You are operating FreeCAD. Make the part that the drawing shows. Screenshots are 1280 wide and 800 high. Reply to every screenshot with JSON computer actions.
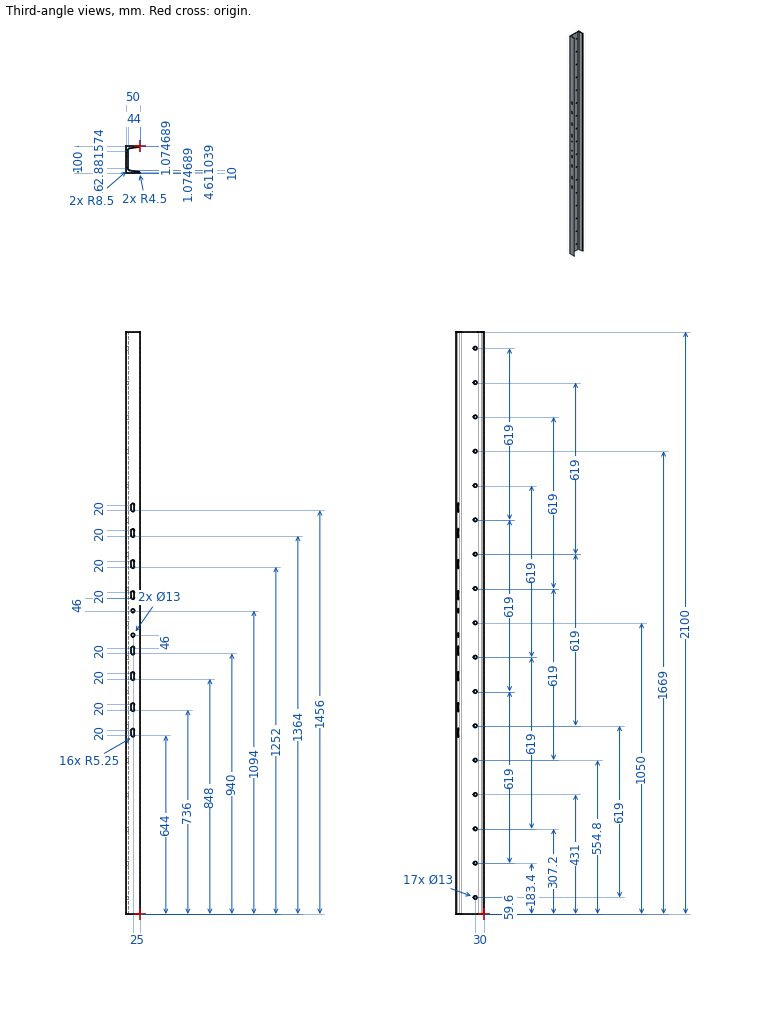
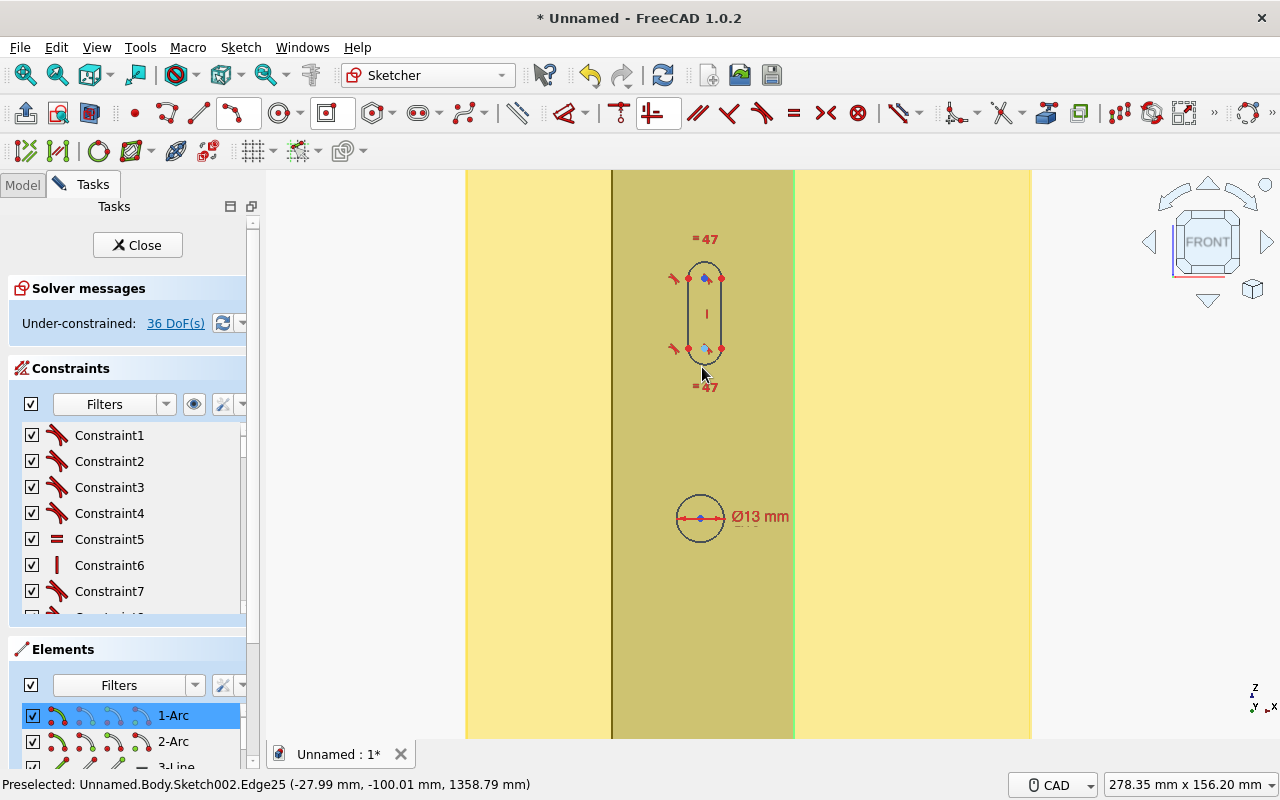
{"action": "left_click", "coordinate": [695, 361]}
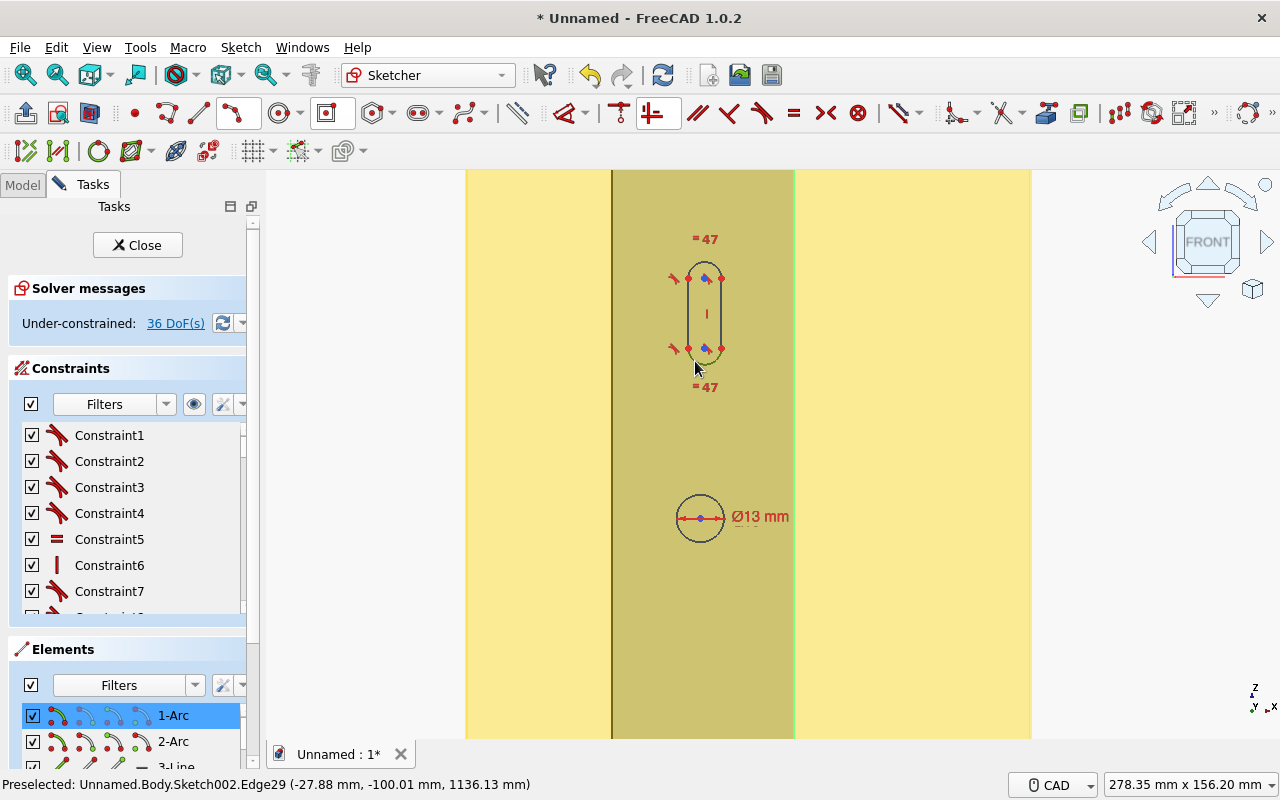
{"action": "left_click", "coordinate": [794, 114]}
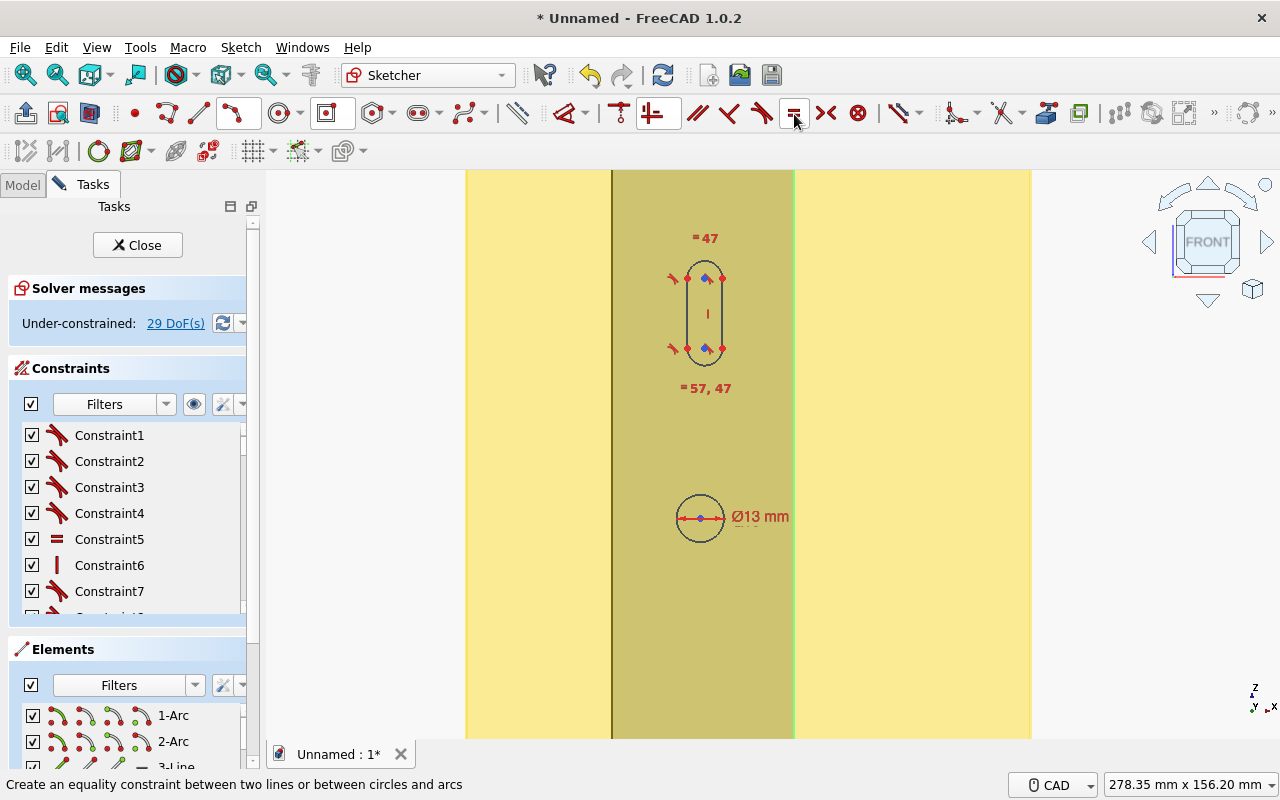
{"action": "left_click", "coordinate": [564, 114]}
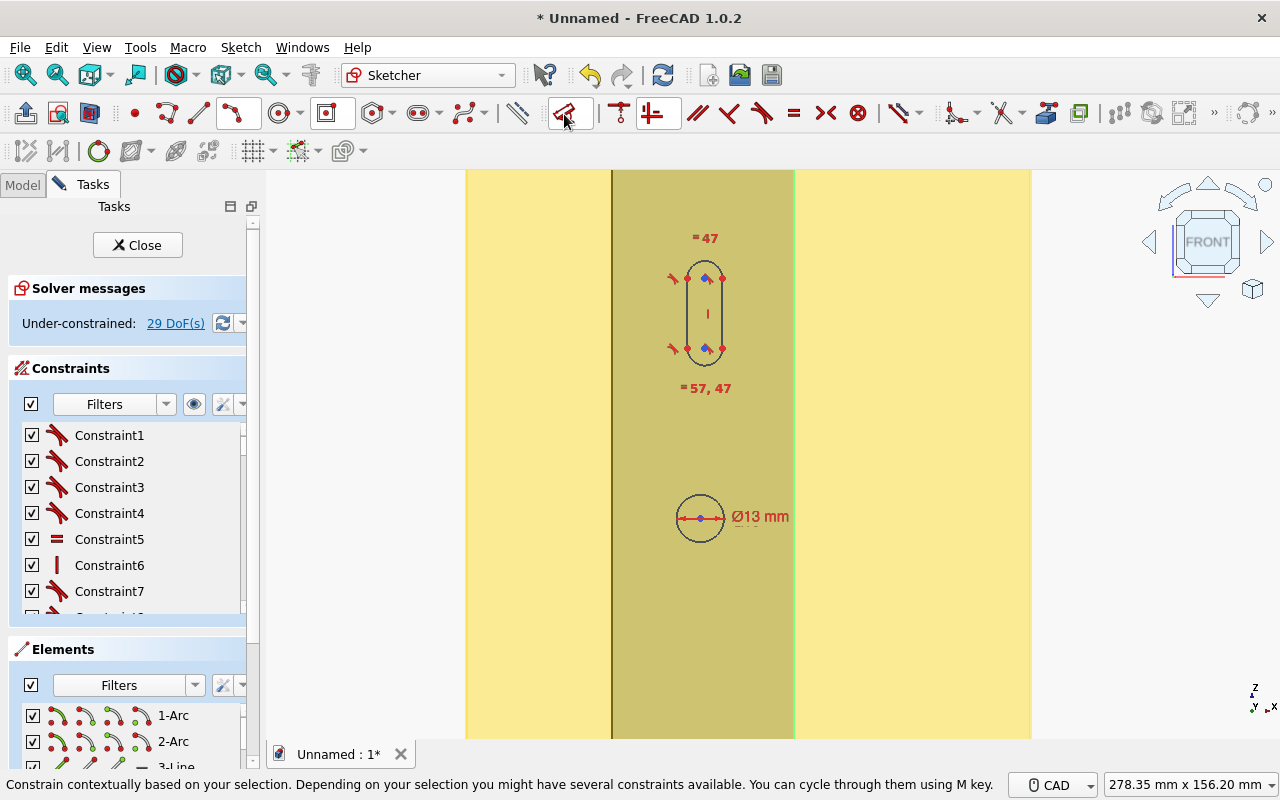
{"action": "scroll", "coordinate": [702, 367], "scroll_direction": "down", "scroll_amount": 14}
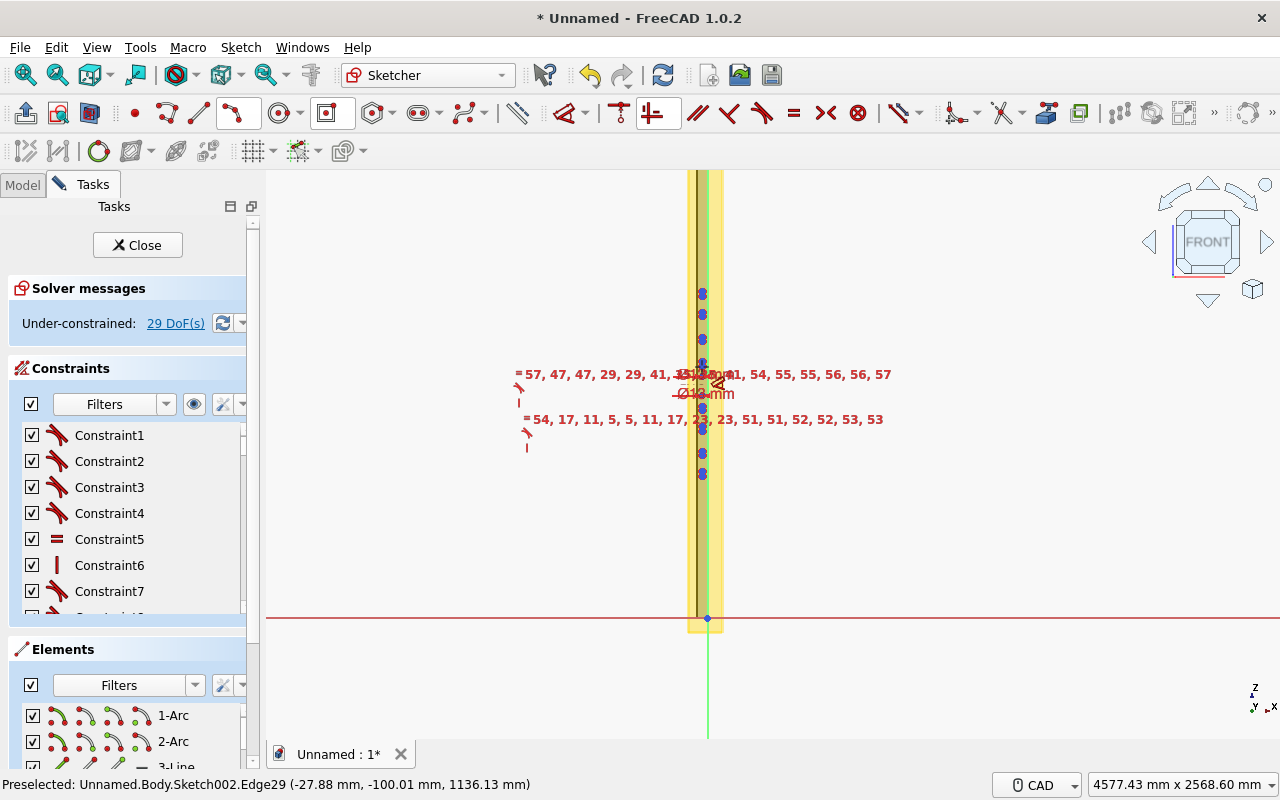
{"action": "scroll", "coordinate": [702, 477], "scroll_direction": "up", "scroll_amount": 18}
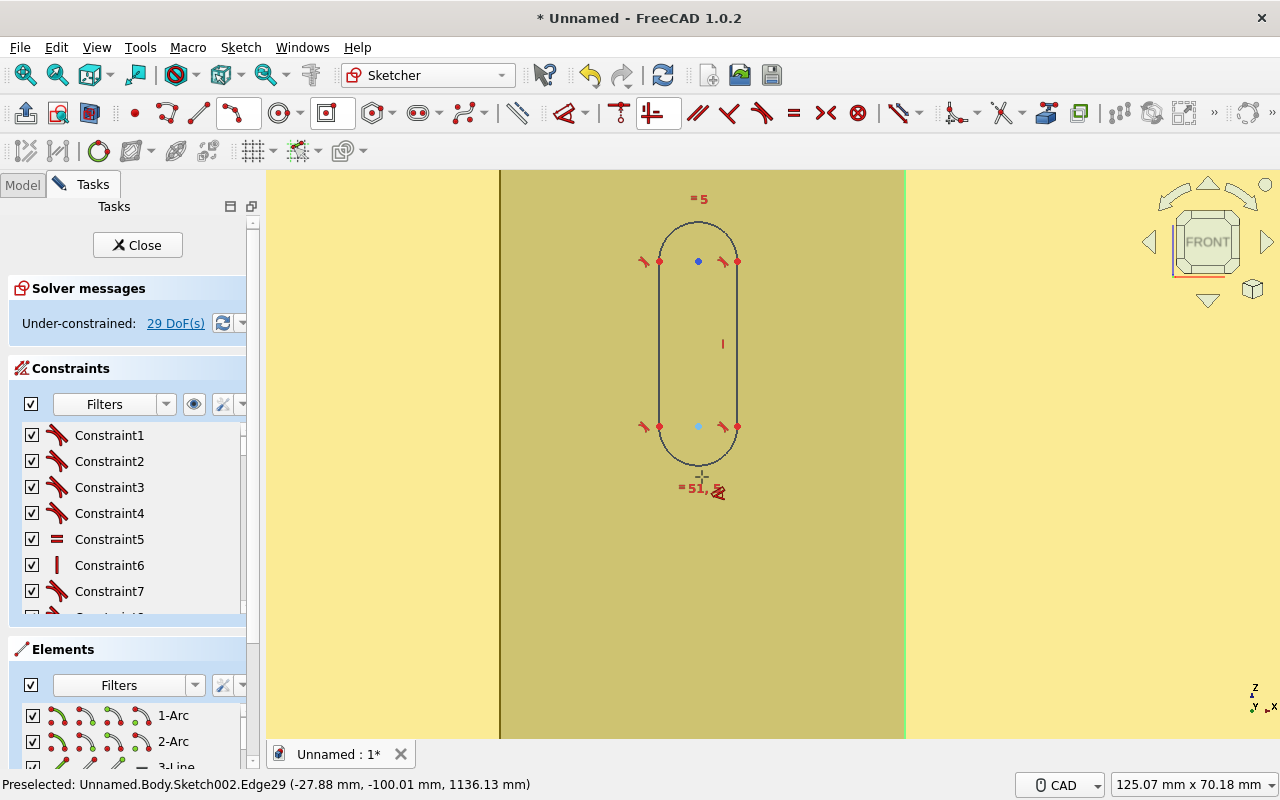
{"action": "left_click", "coordinate": [675, 458]}
{"action": "left_click", "coordinate": [656, 484]}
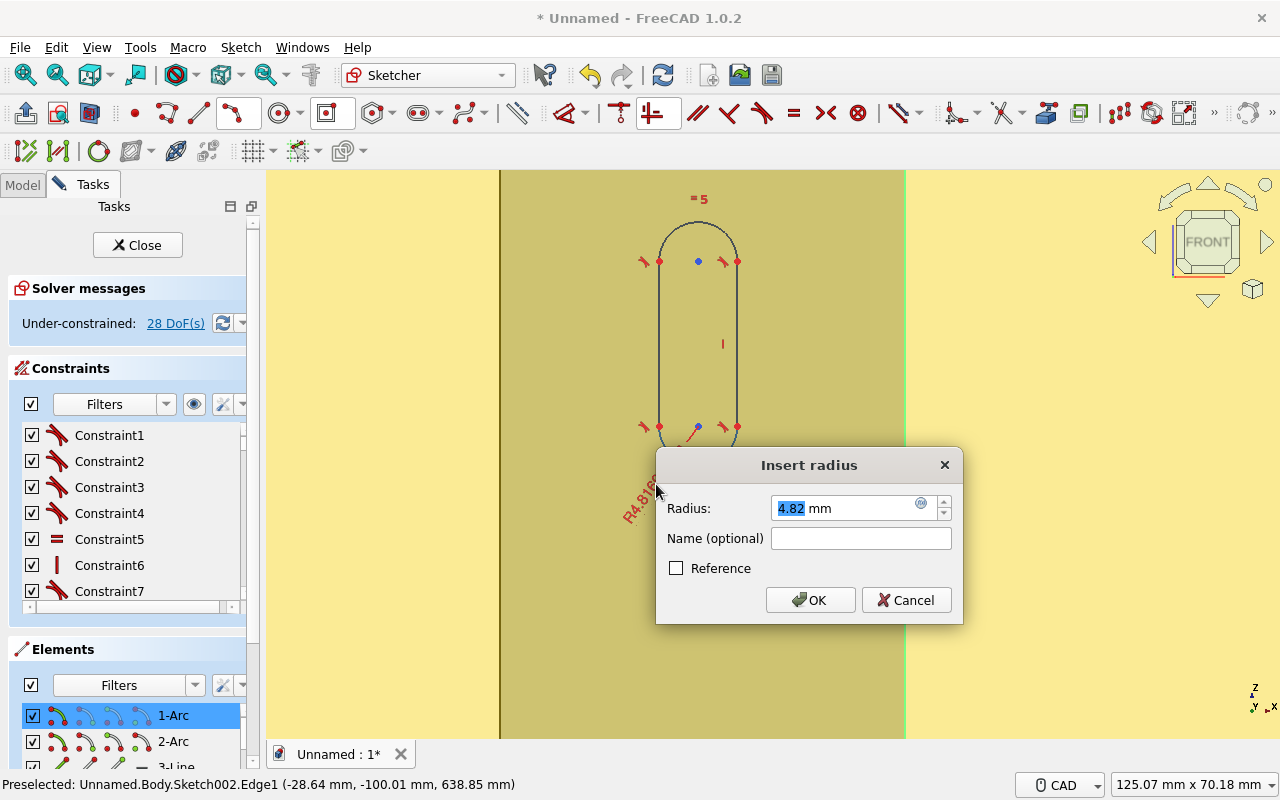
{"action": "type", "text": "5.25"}
{"action": "key", "text": "Return"}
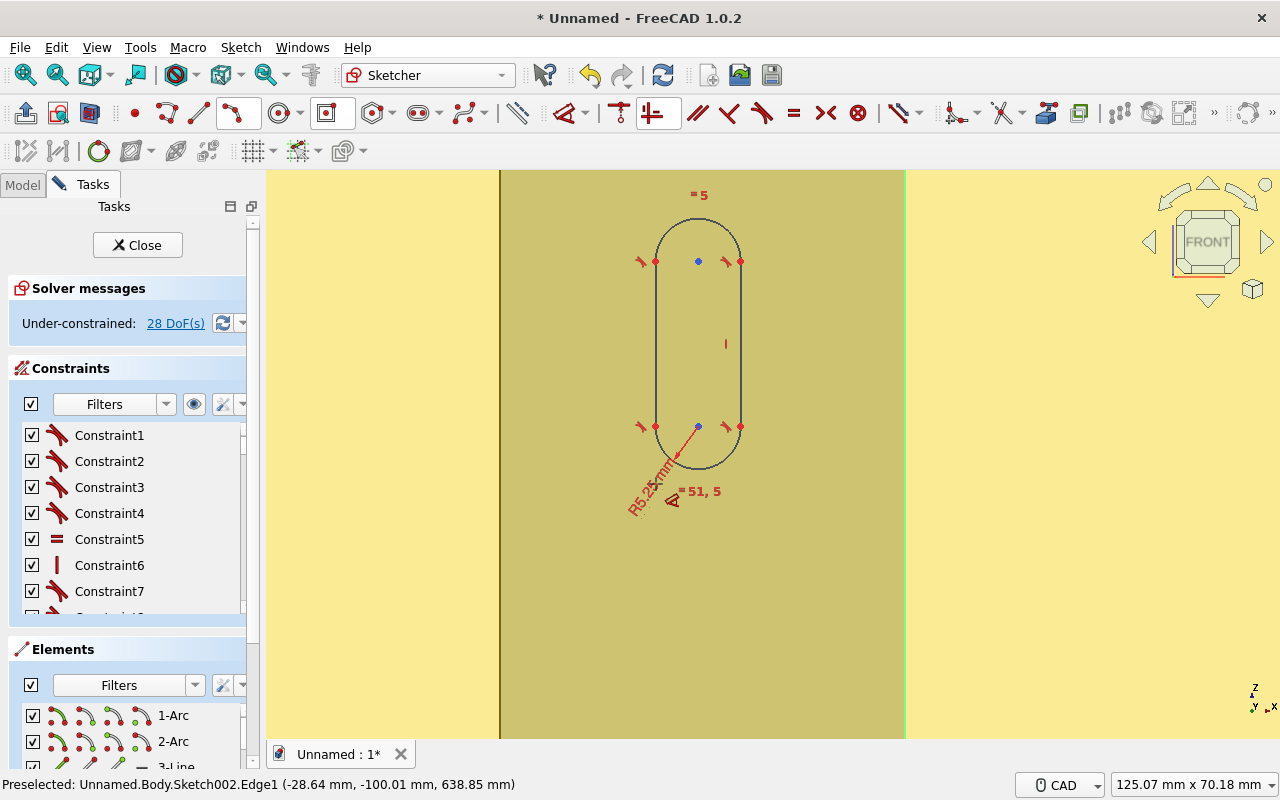
{"action": "scroll", "coordinate": [702, 483], "scroll_direction": "down", "scroll_amount": 17}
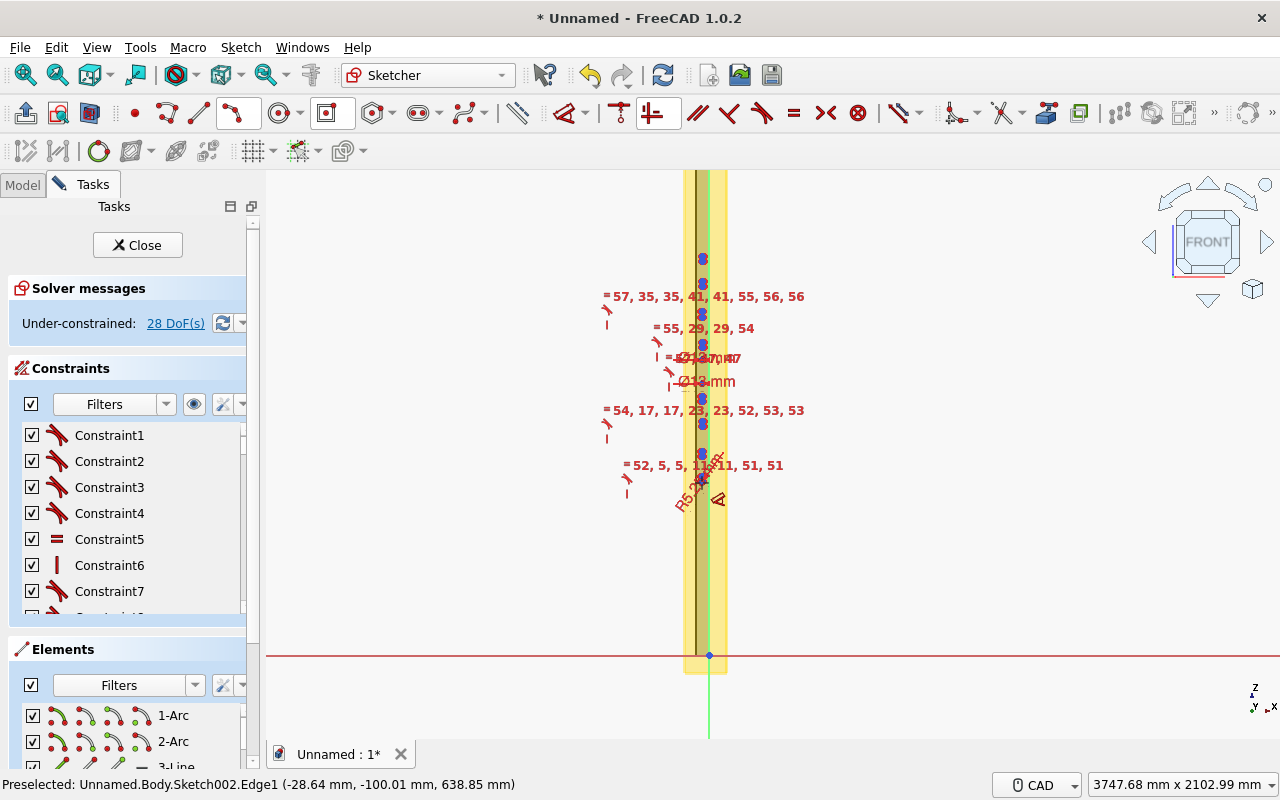
{"action": "scroll", "coordinate": [701, 480], "scroll_direction": "up", "scroll_amount": 11}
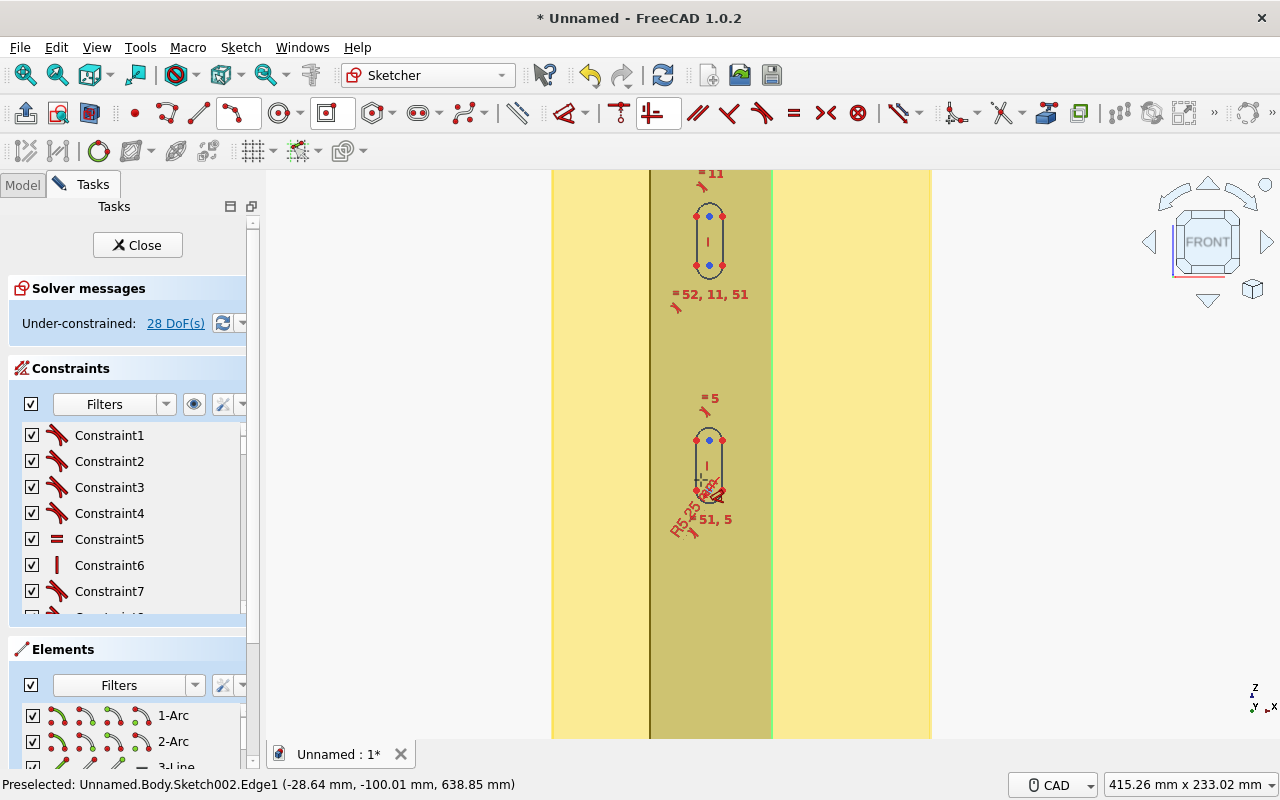
{"action": "left_click", "coordinate": [696, 476]}
{"action": "left_click", "coordinate": [662, 466]}